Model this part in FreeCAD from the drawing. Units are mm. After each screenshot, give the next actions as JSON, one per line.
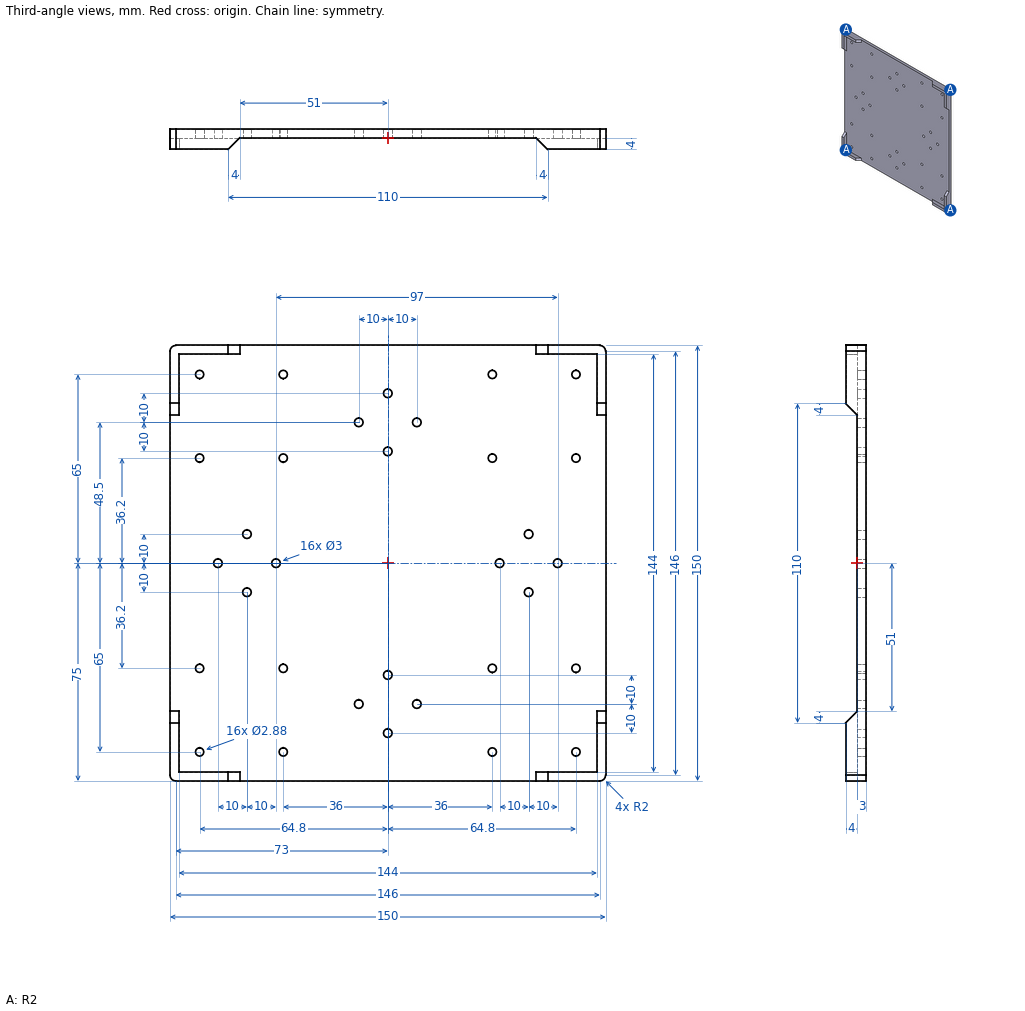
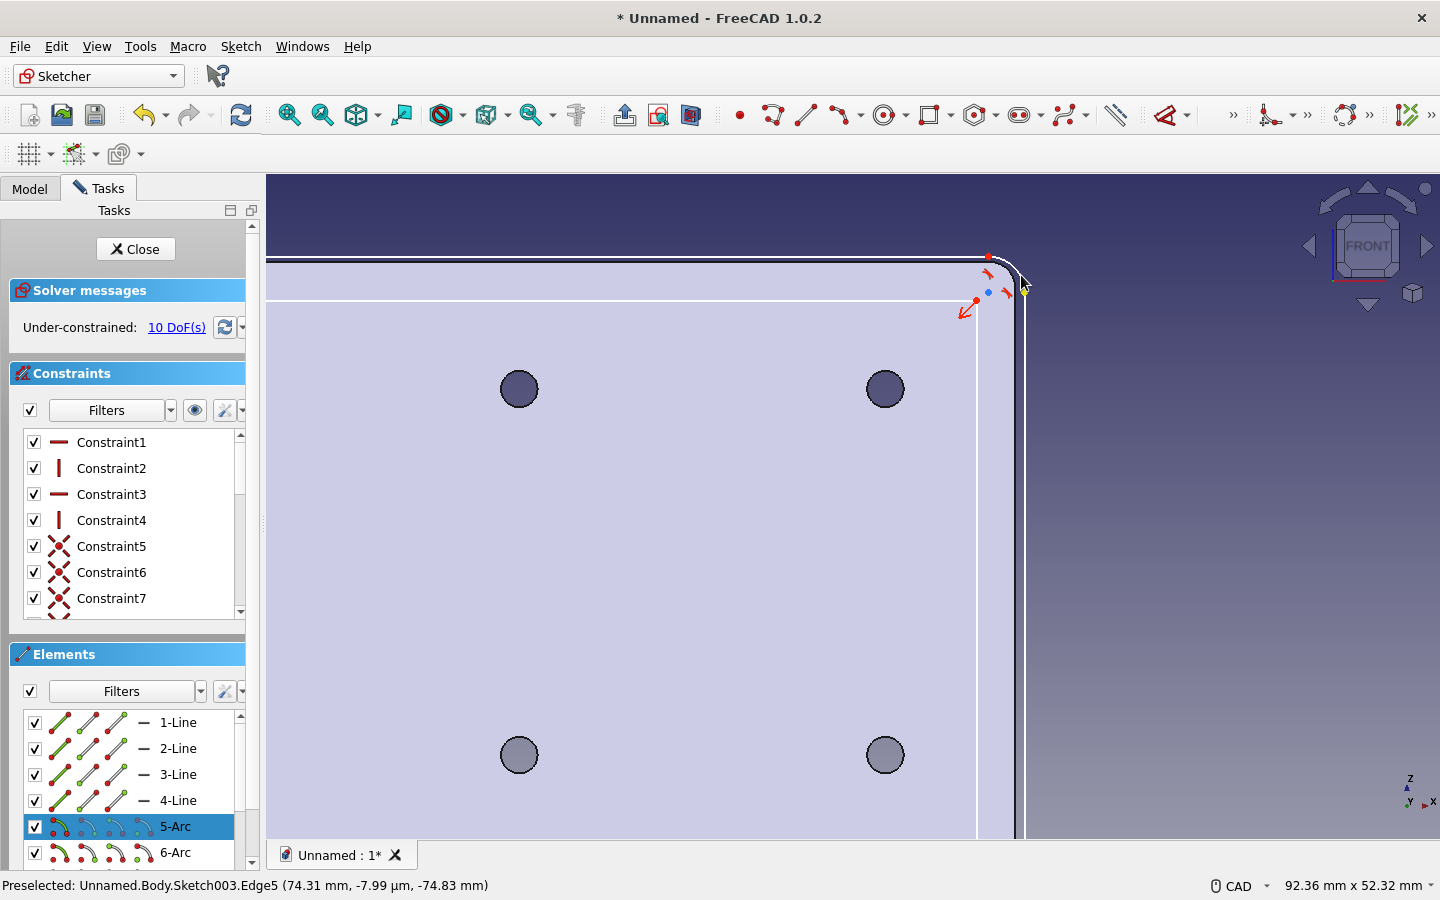
{"action": "left_click", "coordinate": [1021, 276]}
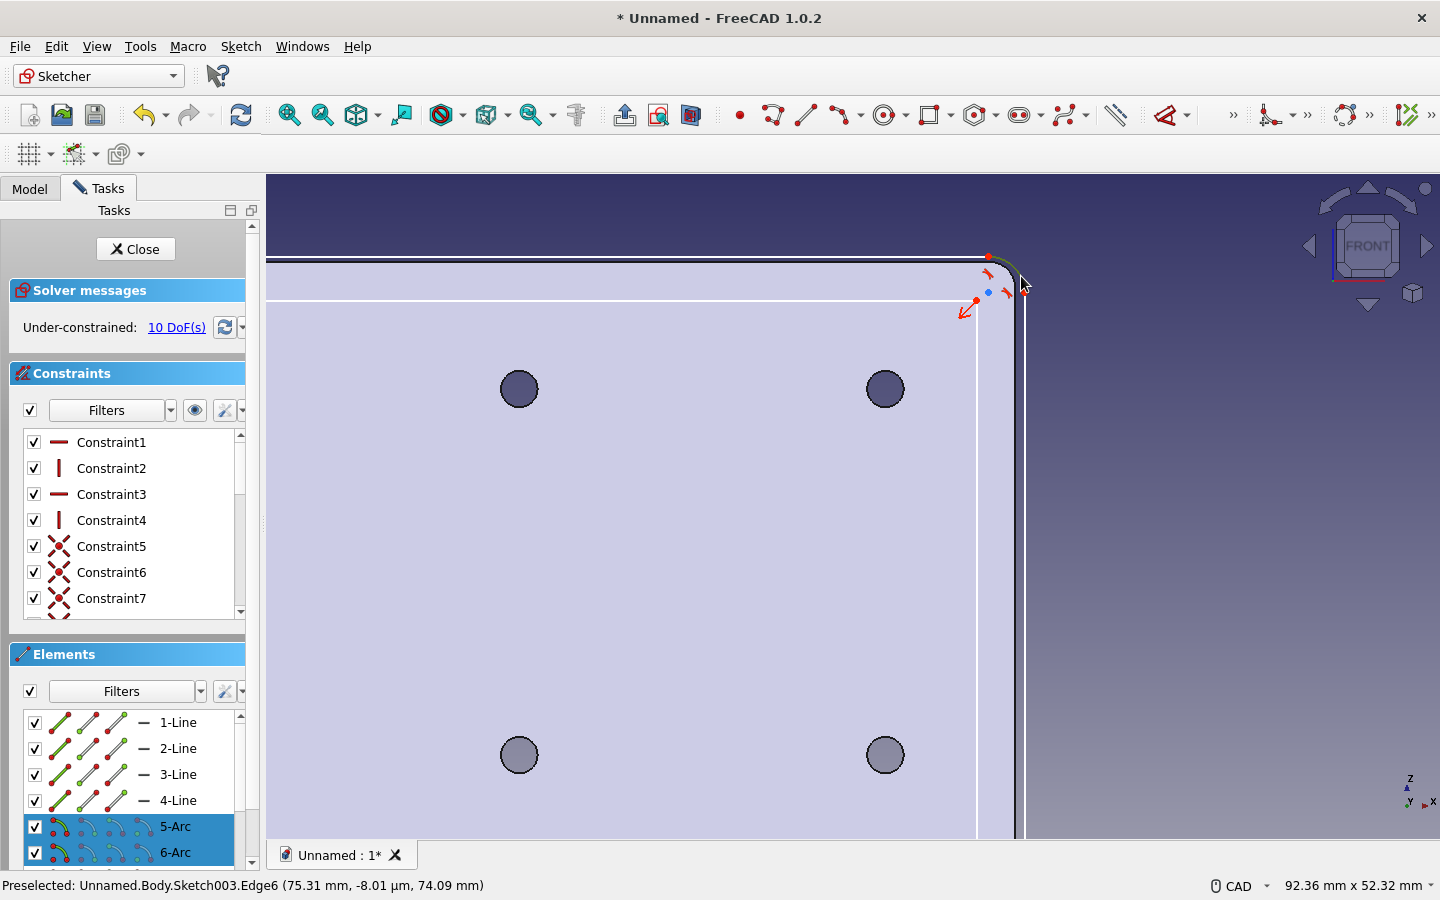
{"action": "scroll", "coordinate": [1021, 275], "scroll_direction": "down", "scroll_amount": 7}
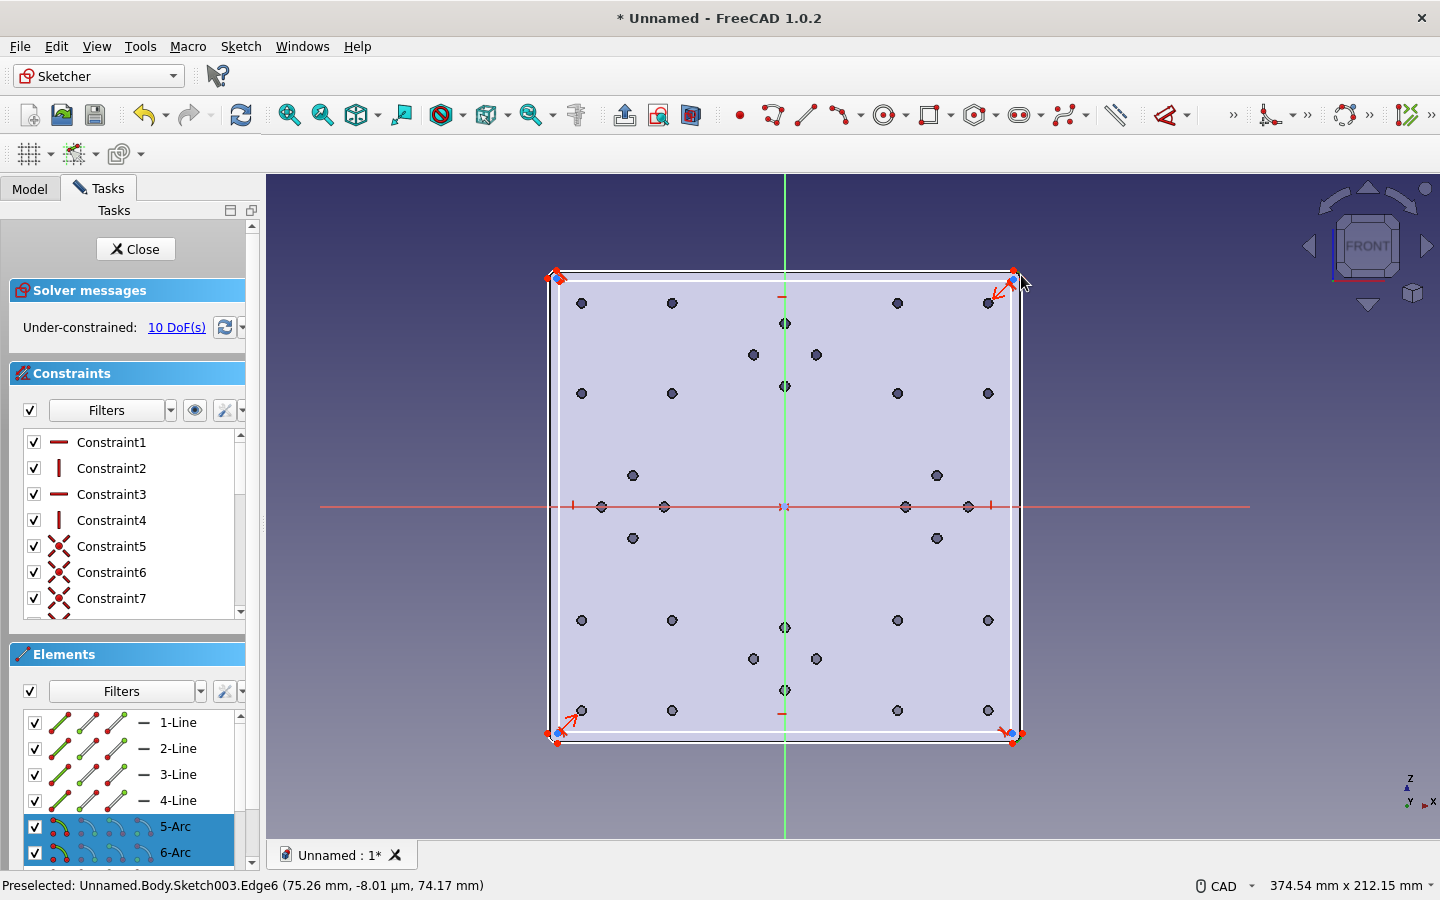
{"action": "scroll", "coordinate": [552, 272], "scroll_direction": "up", "scroll_amount": 7}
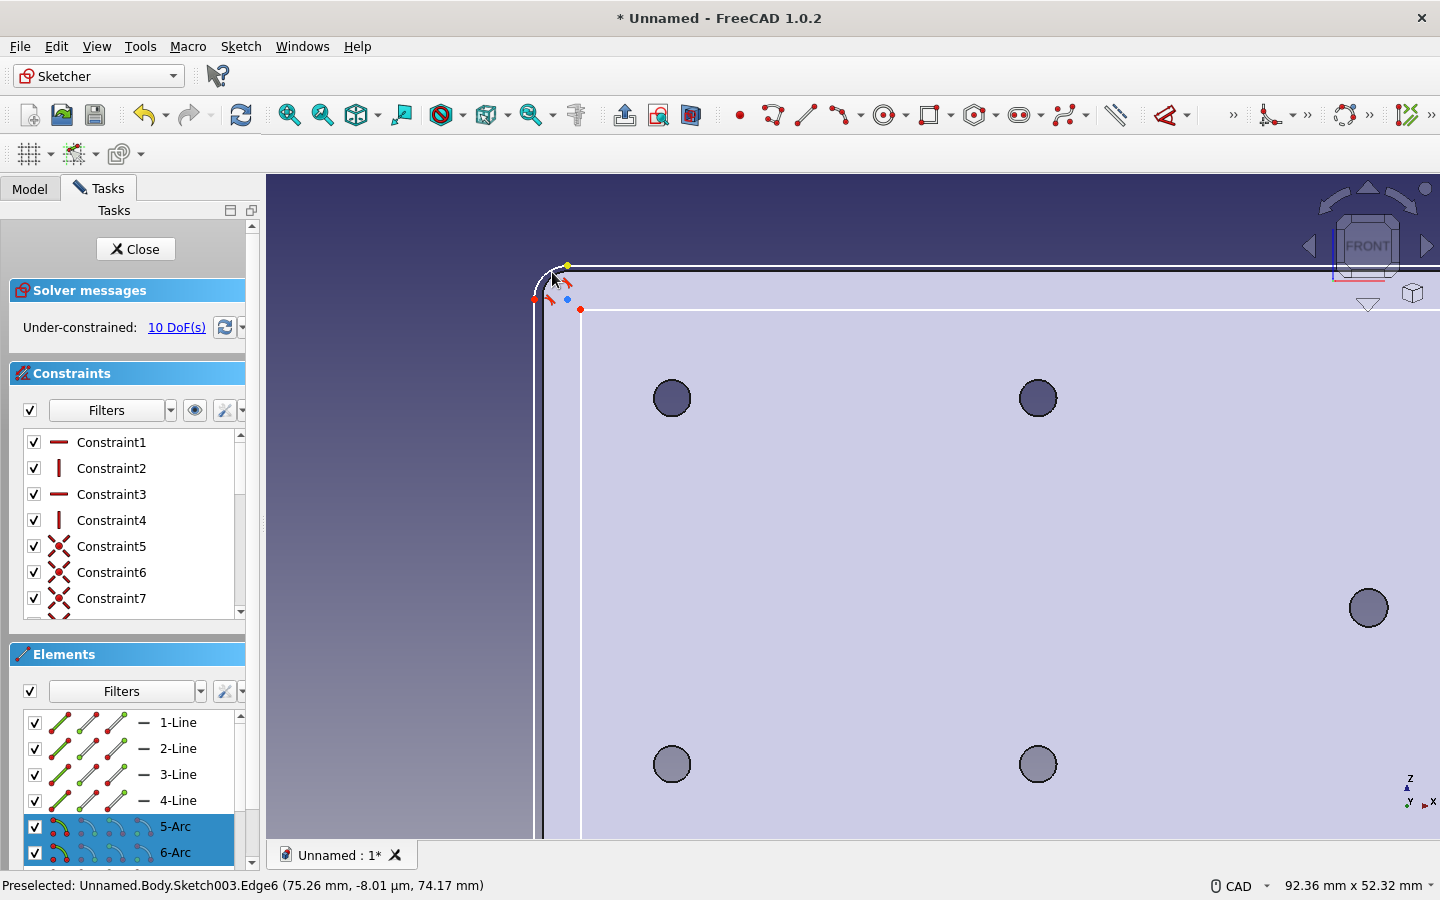
{"action": "left_click", "coordinate": [552, 270]}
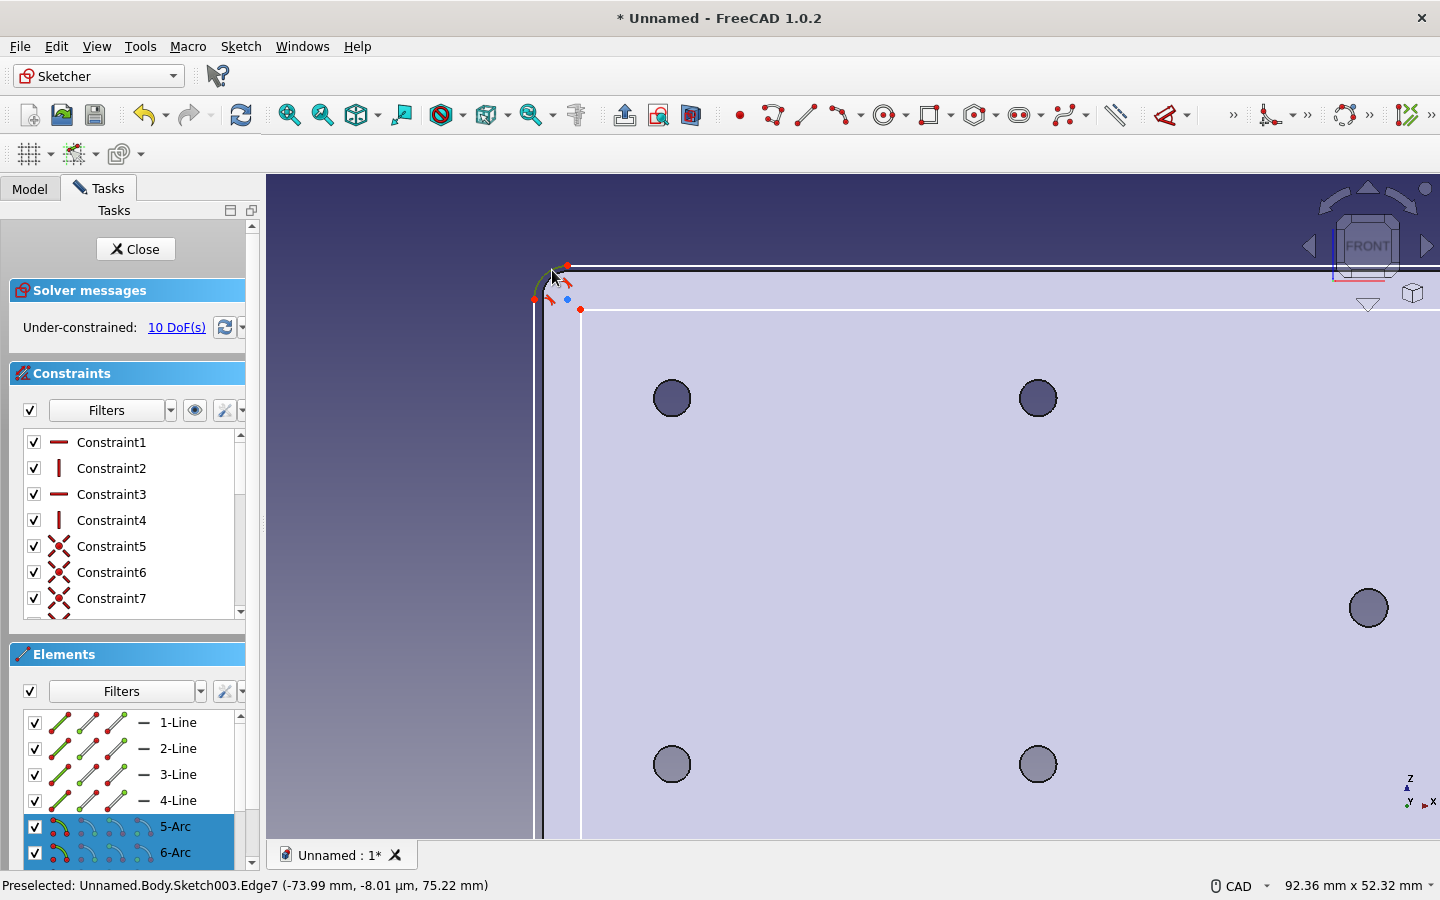
{"action": "scroll", "coordinate": [552, 272], "scroll_direction": "down", "scroll_amount": 7}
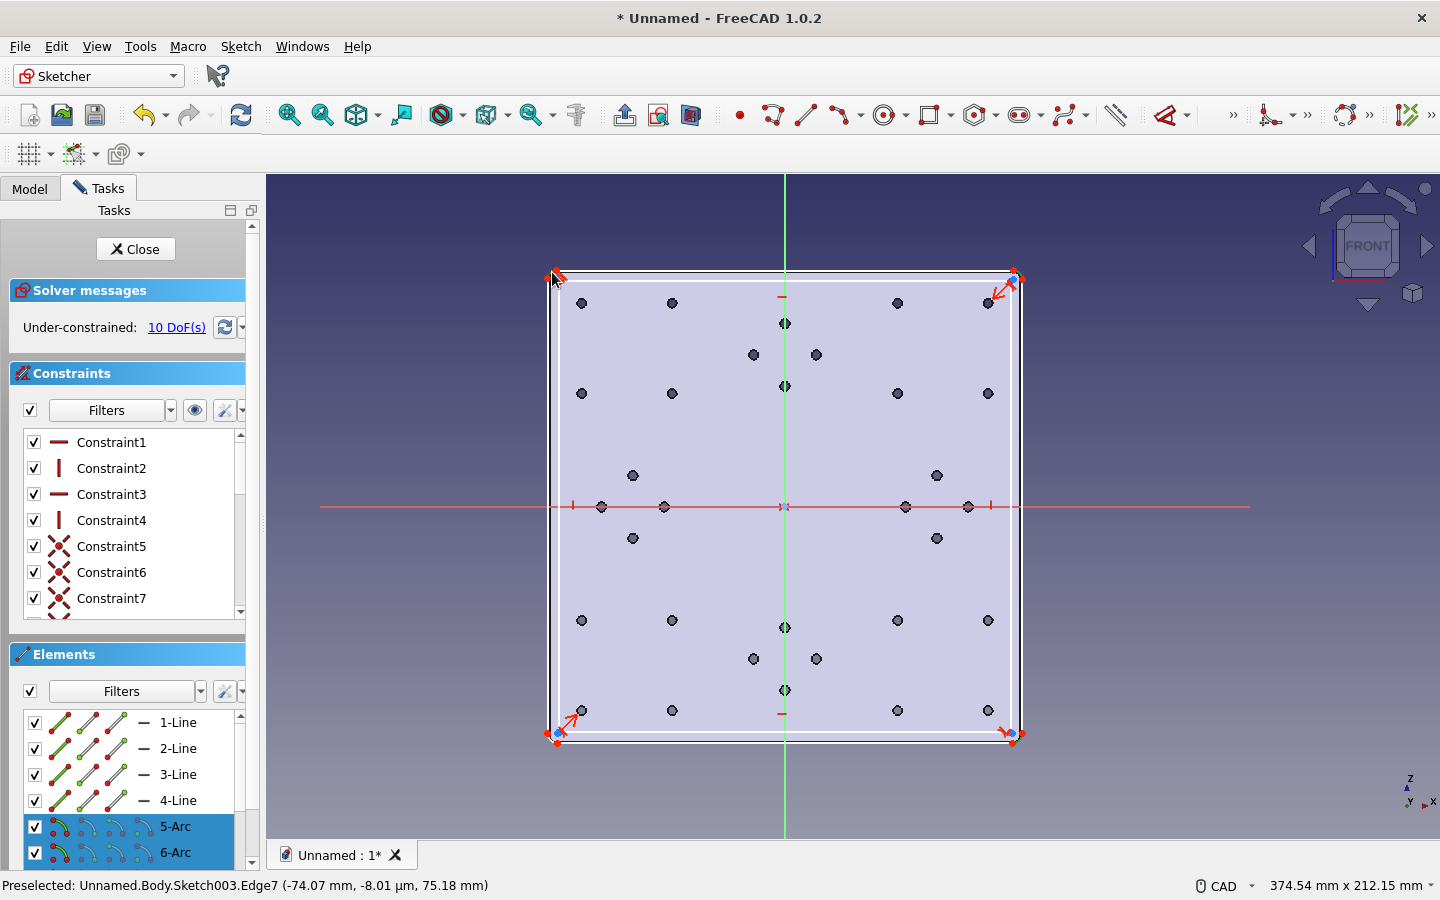
{"action": "scroll", "coordinate": [549, 738], "scroll_direction": "up", "scroll_amount": 6}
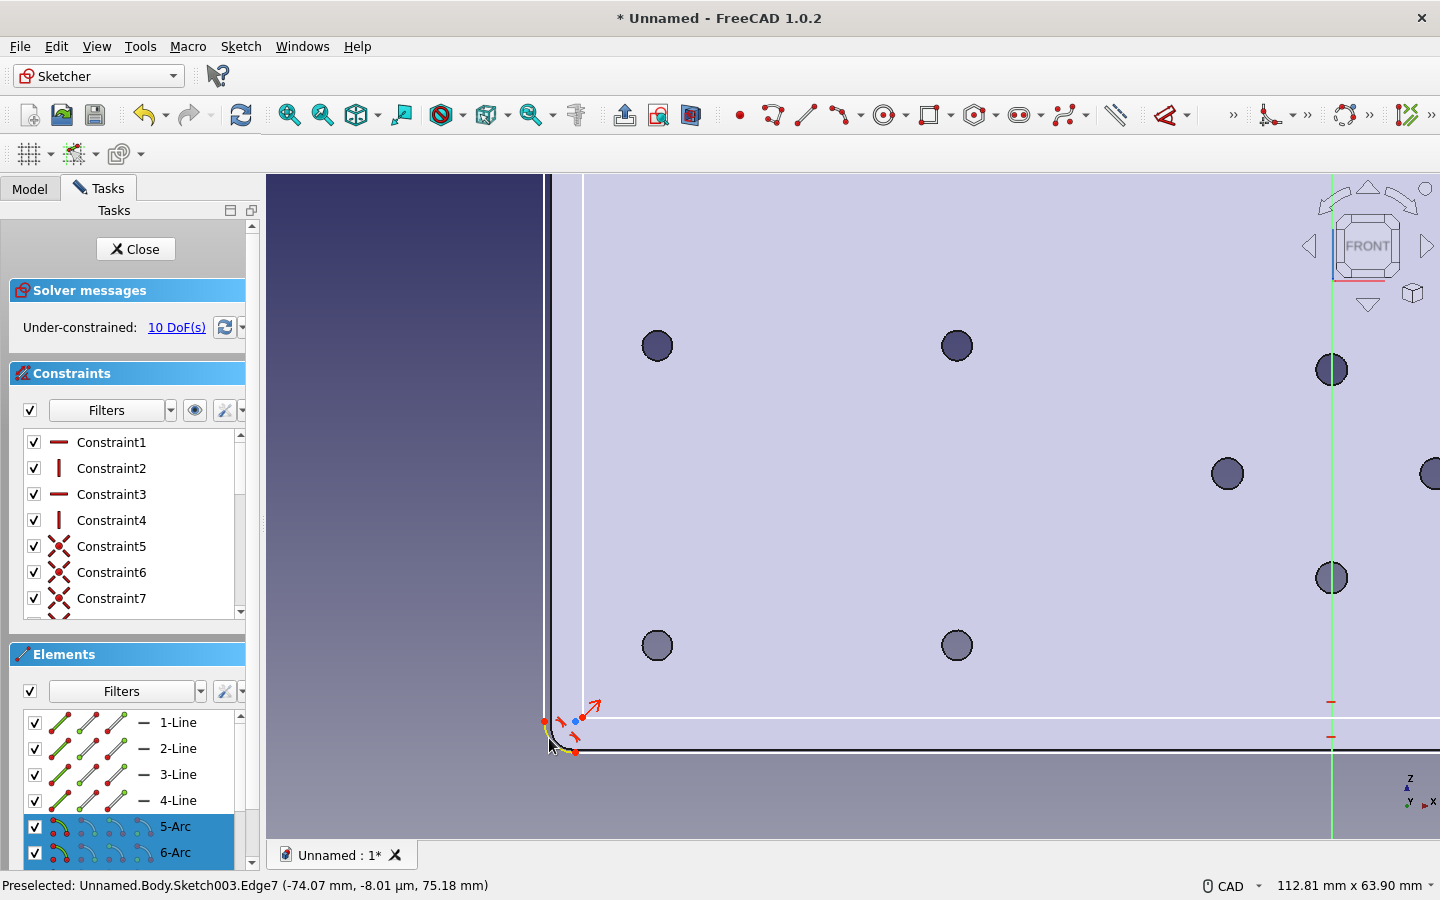
{"action": "left_click", "coordinate": [548, 736]}